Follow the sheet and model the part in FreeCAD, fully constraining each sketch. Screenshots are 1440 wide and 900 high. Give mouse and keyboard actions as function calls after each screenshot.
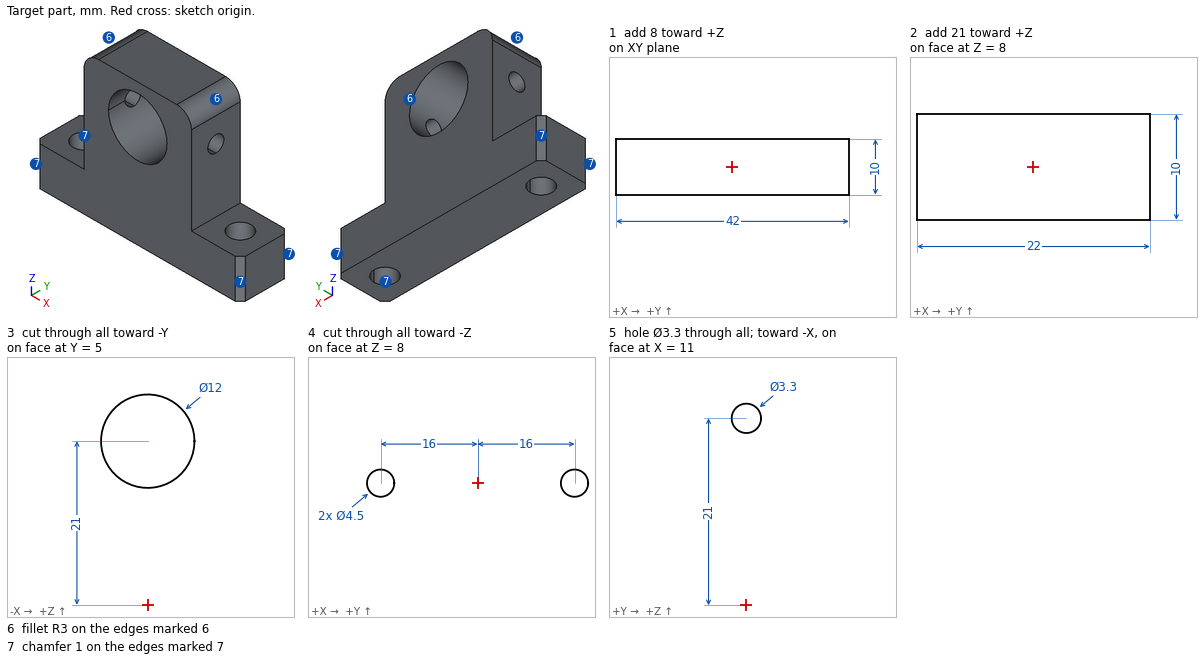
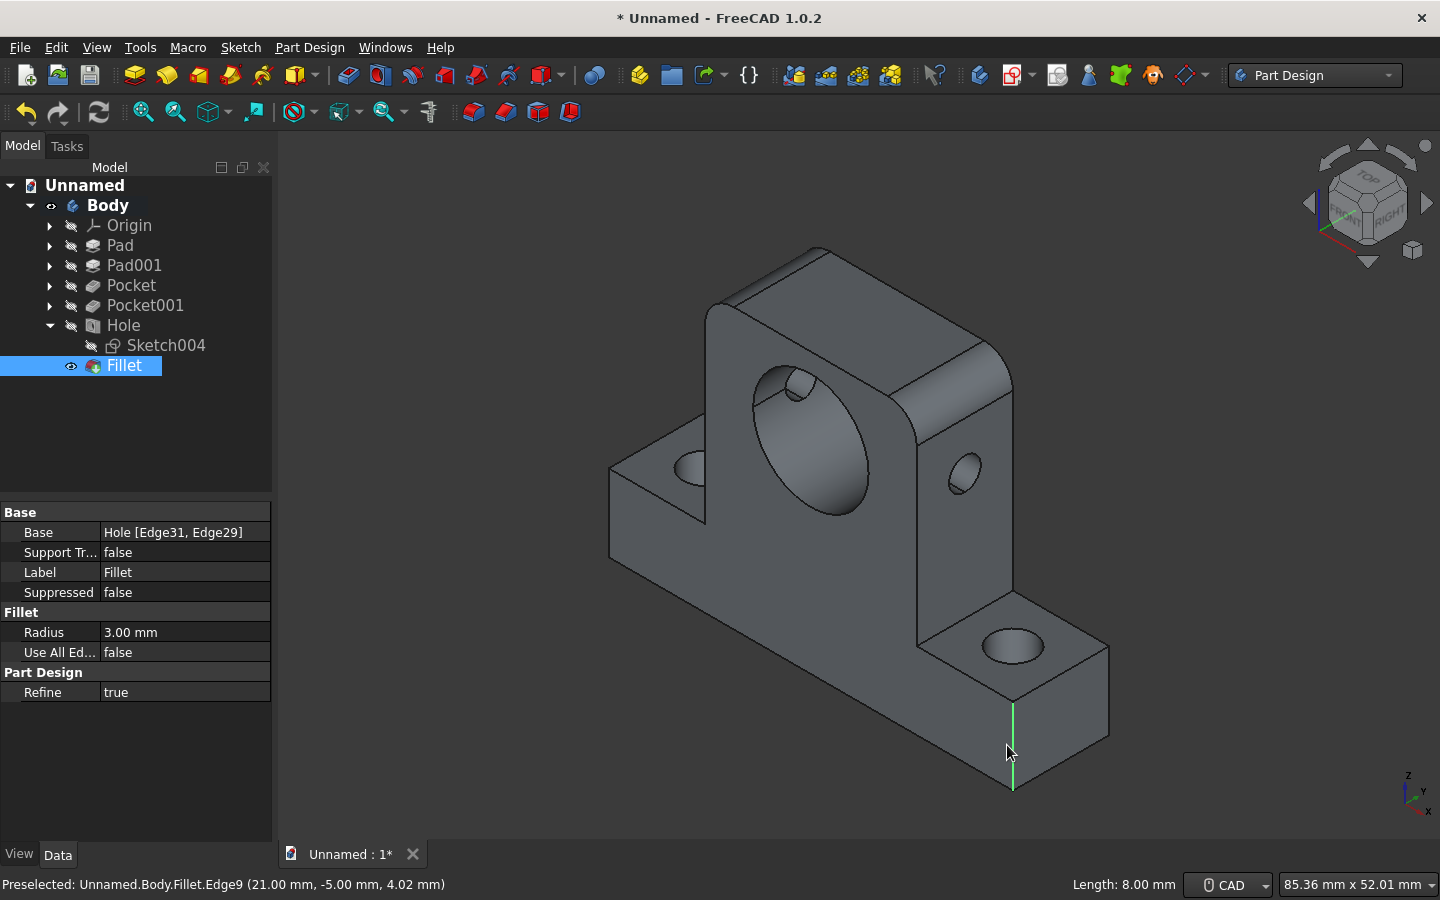
key(2)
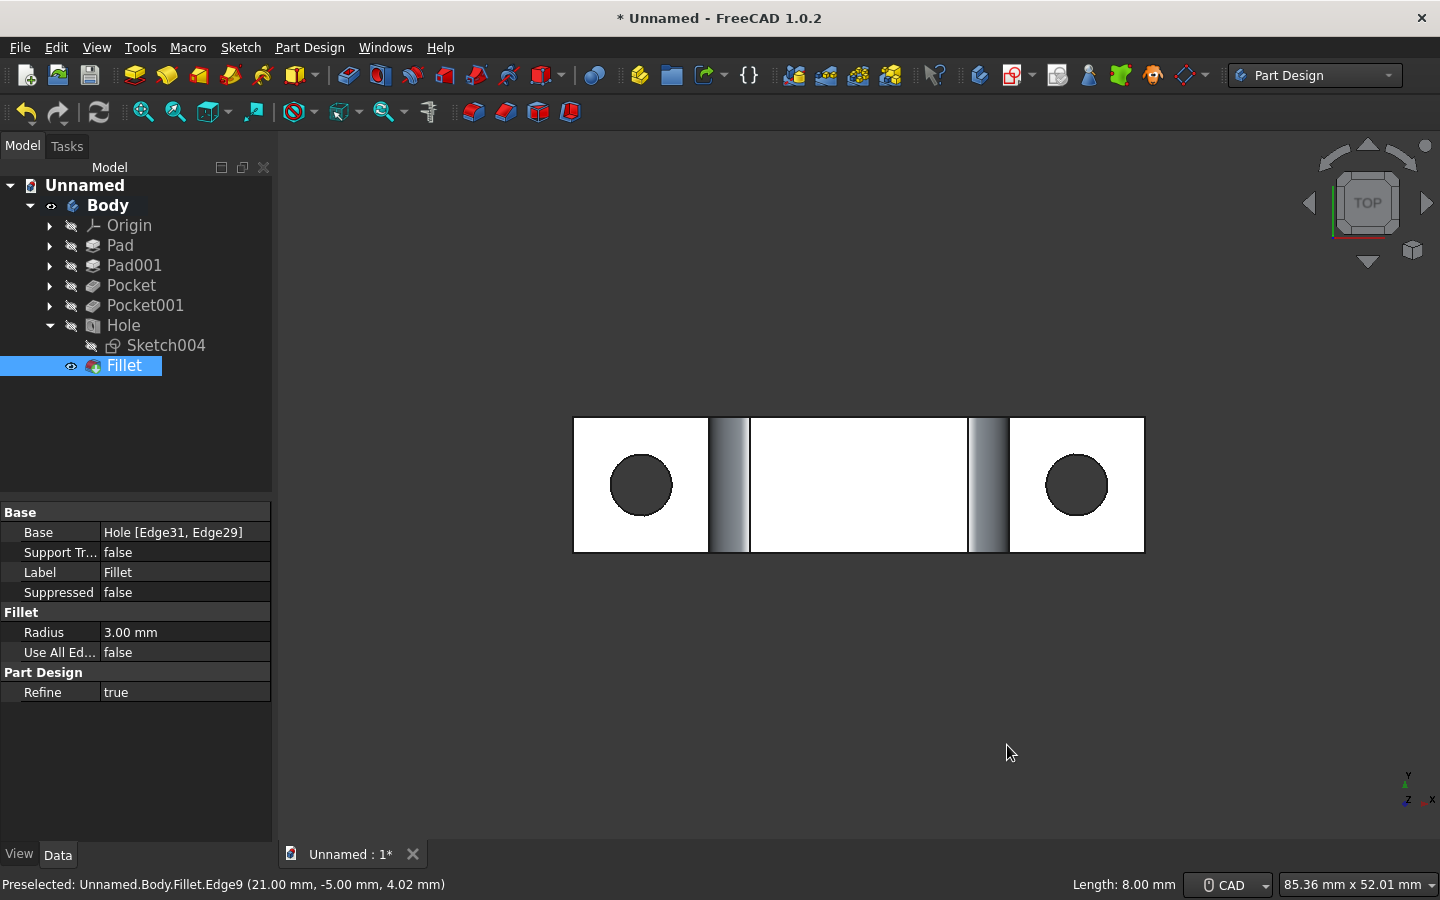
key(1)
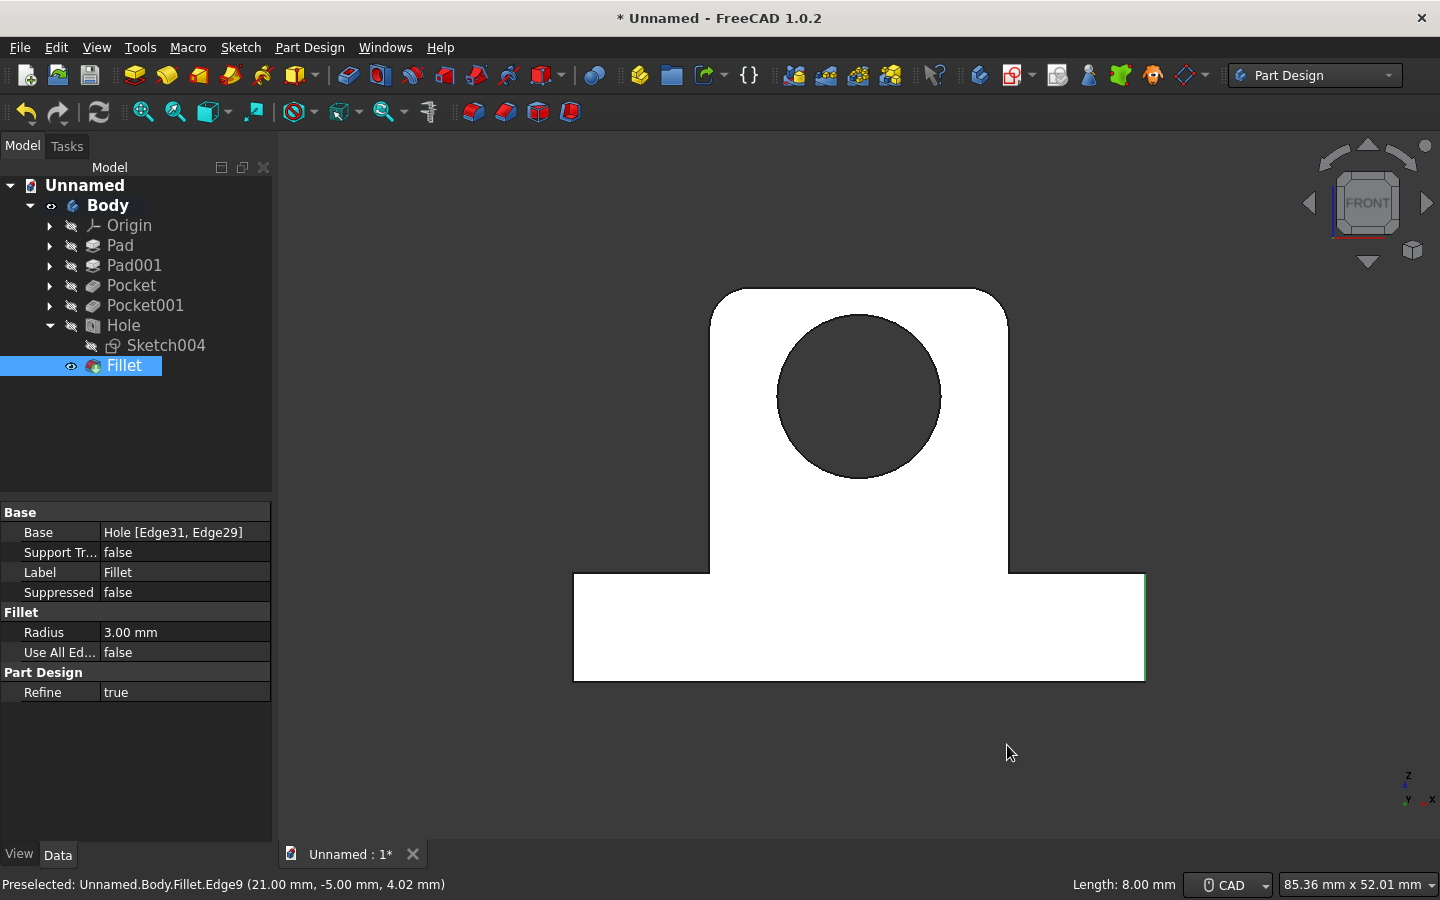
click(573, 627, ctrl)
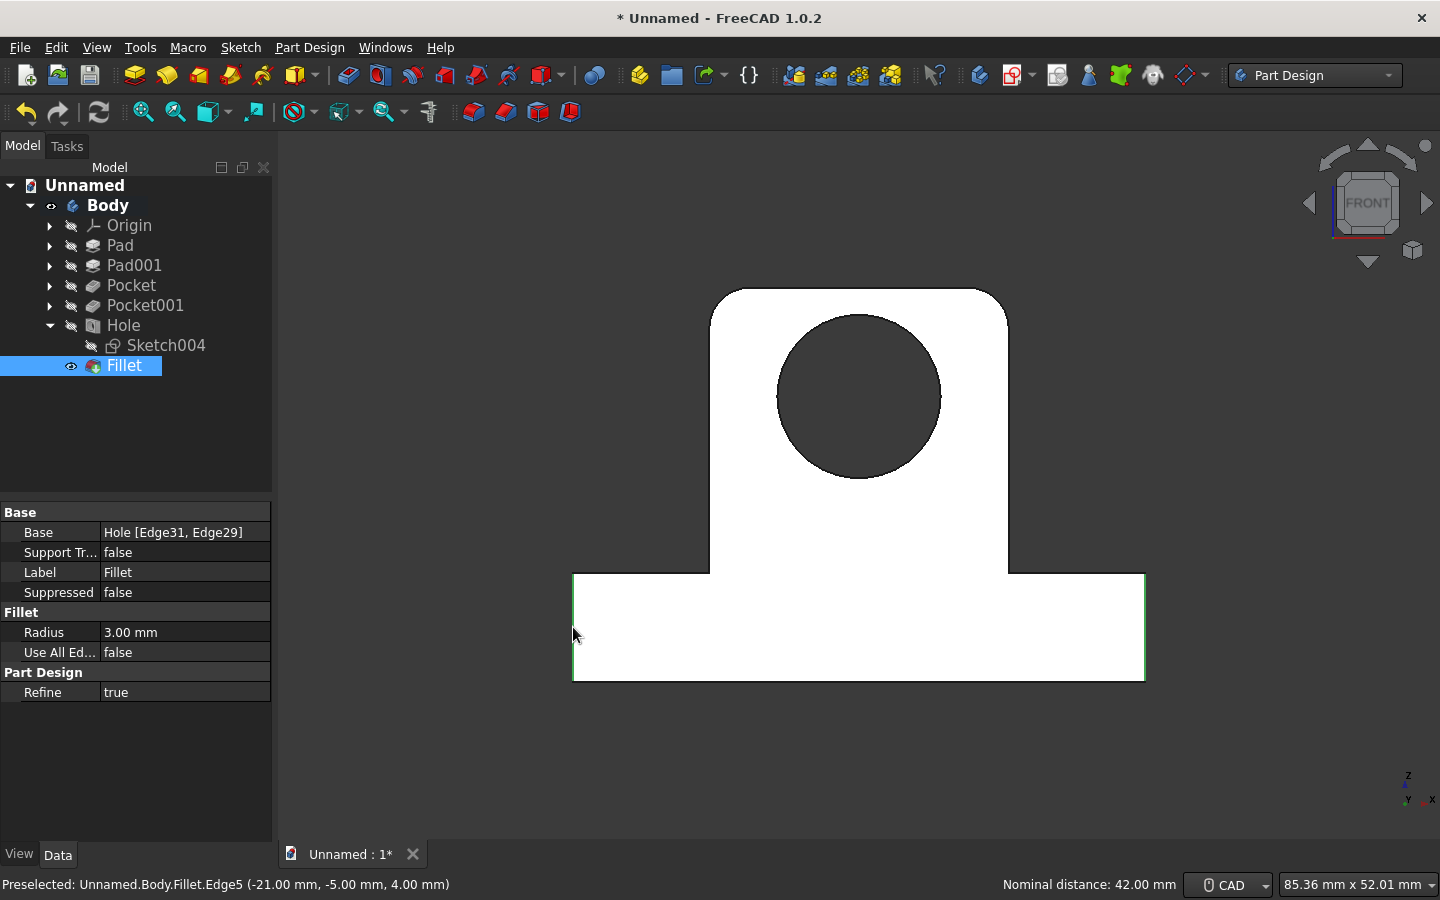
key(3)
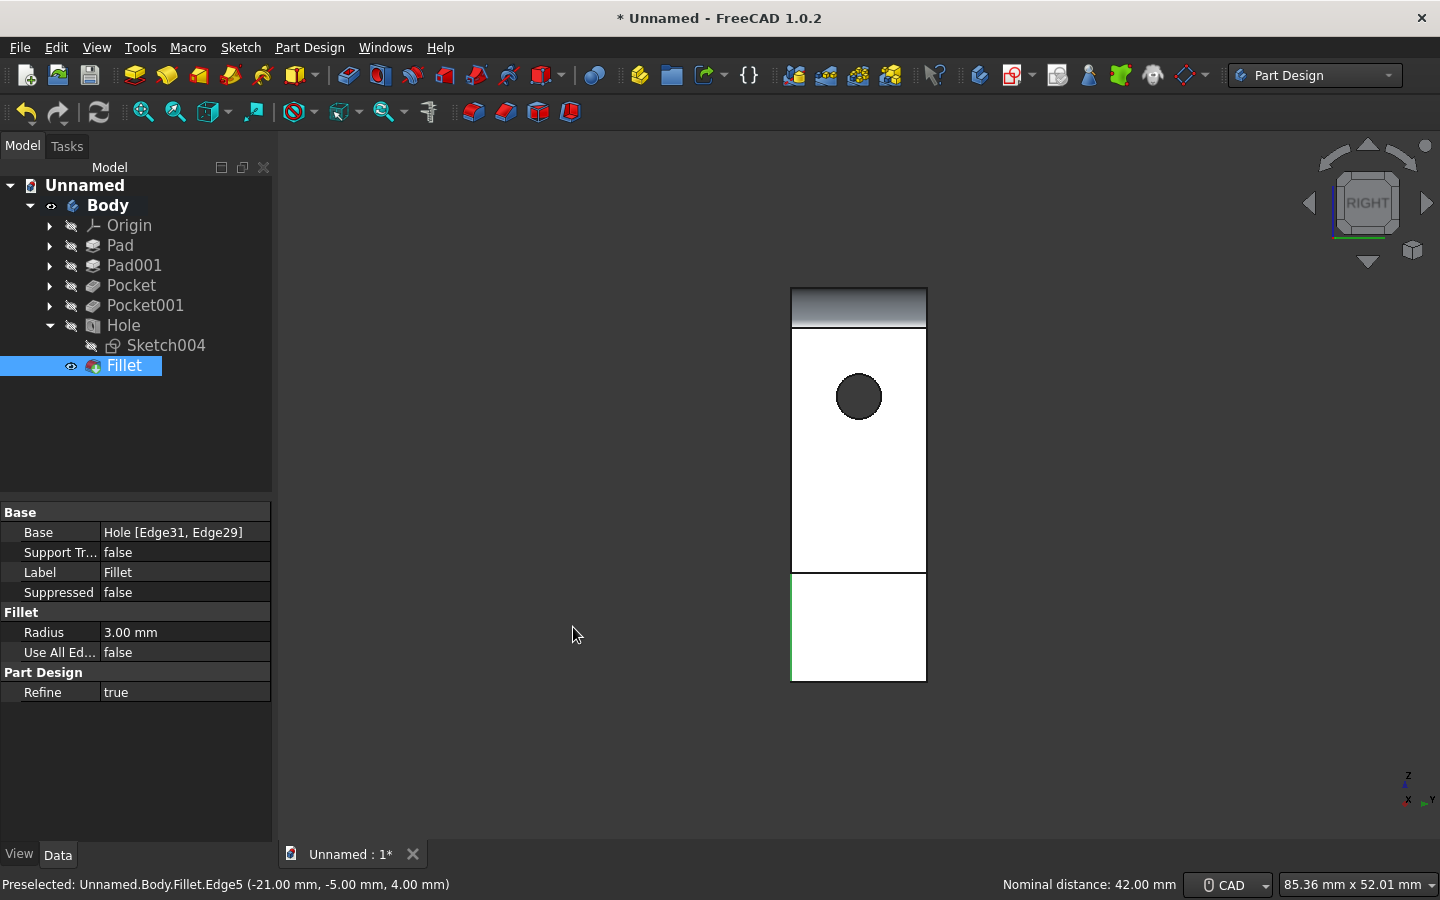
click(927, 627, ctrl)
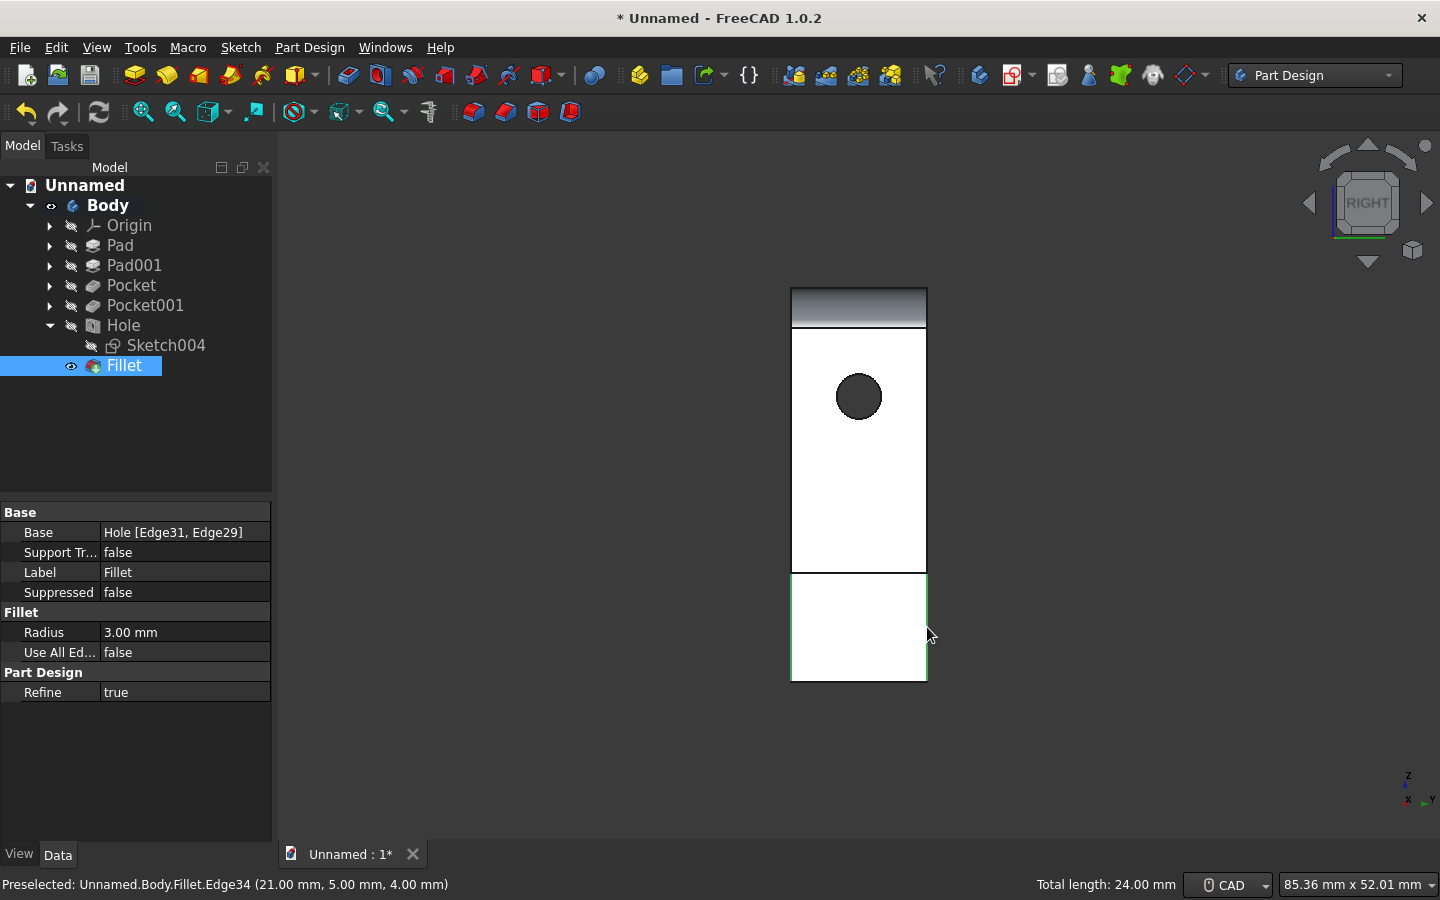
key(5)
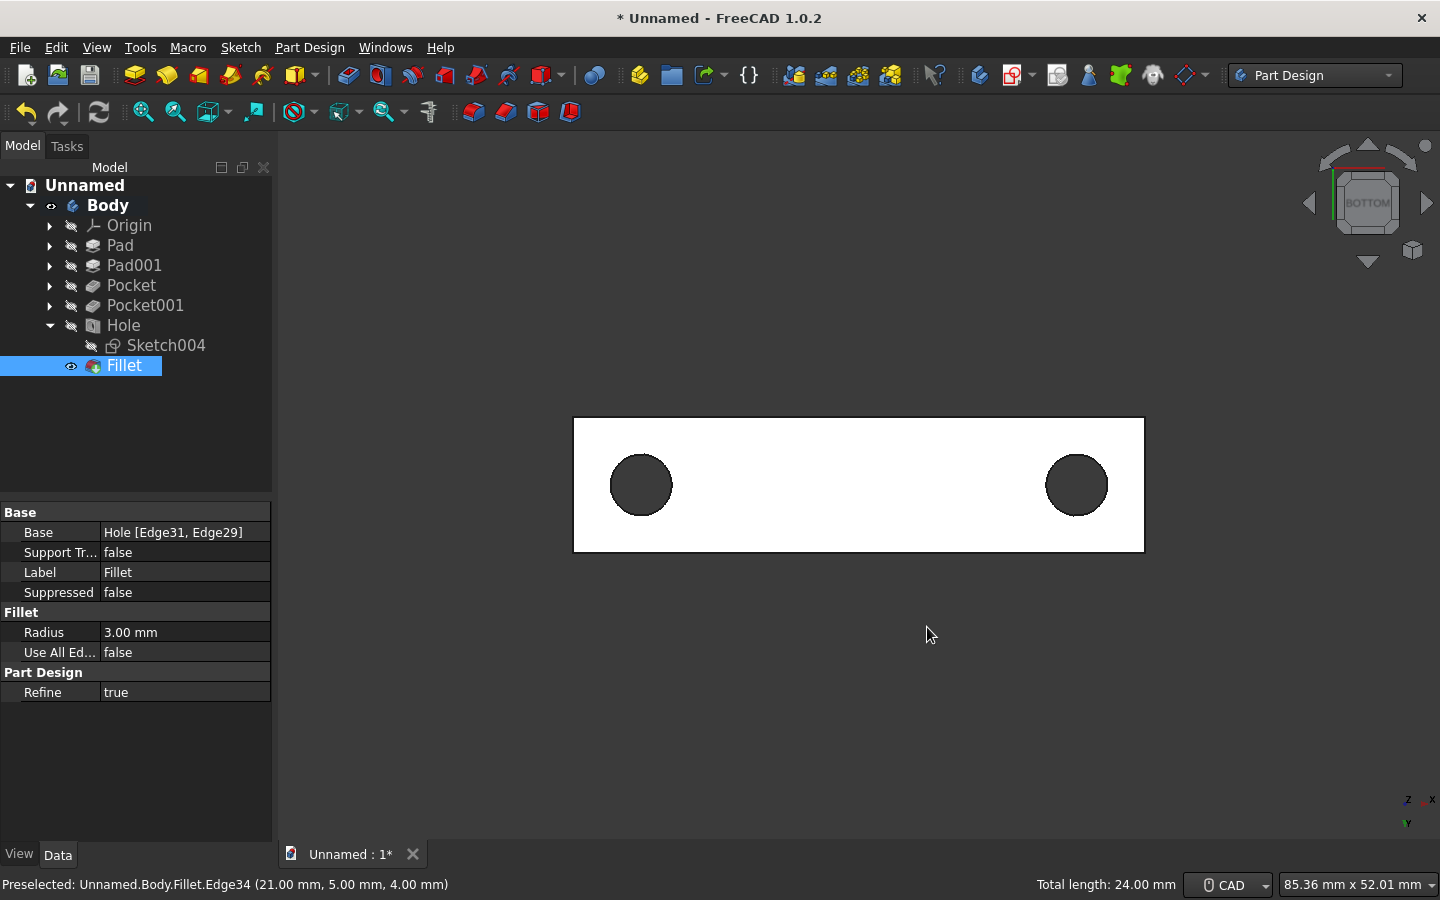
key(4)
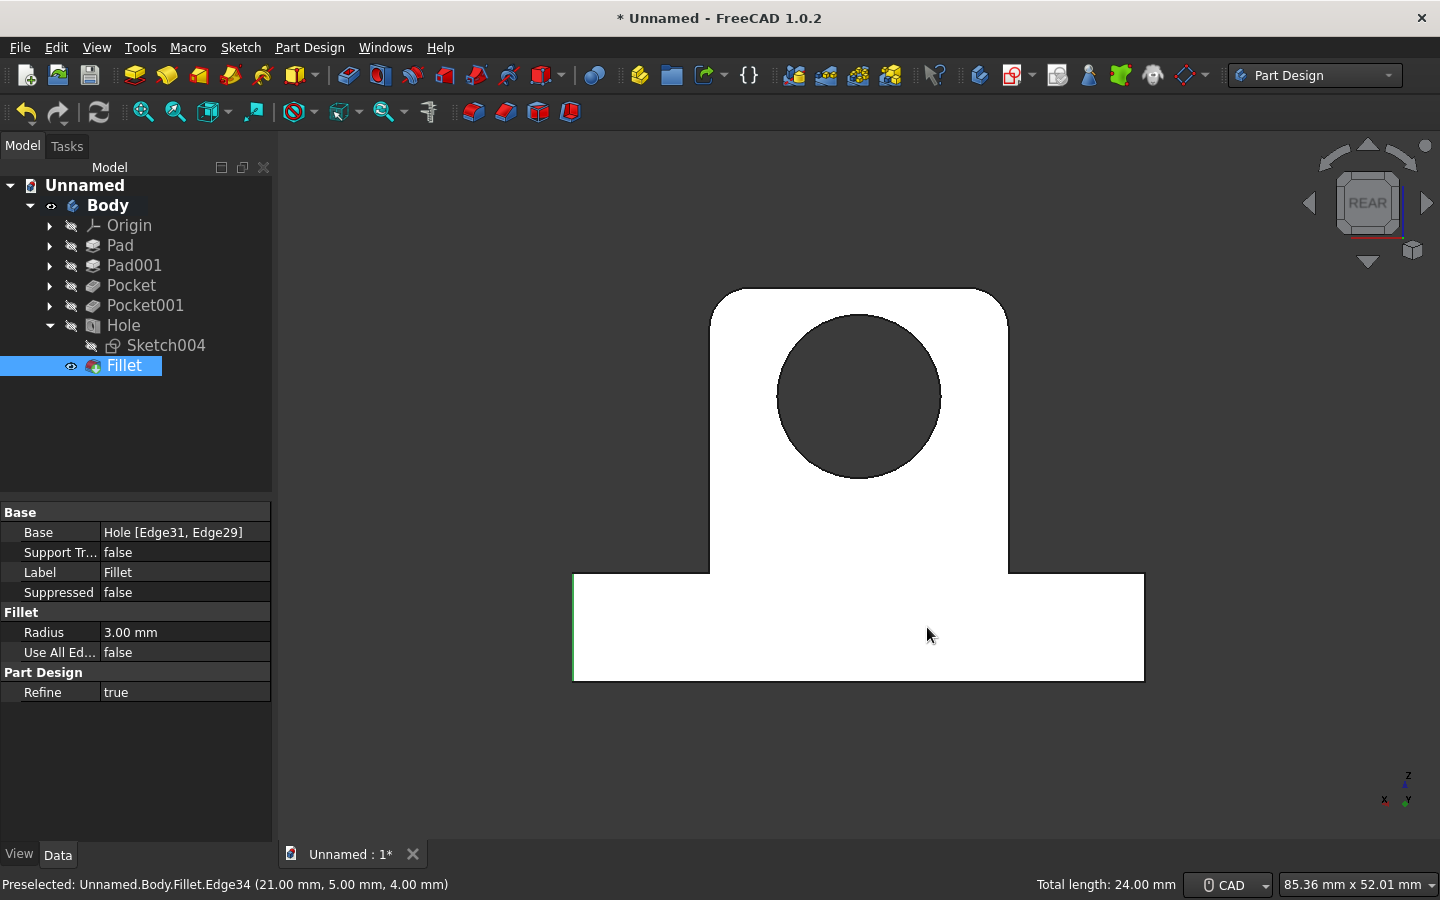
click(1145, 627, ctrl)